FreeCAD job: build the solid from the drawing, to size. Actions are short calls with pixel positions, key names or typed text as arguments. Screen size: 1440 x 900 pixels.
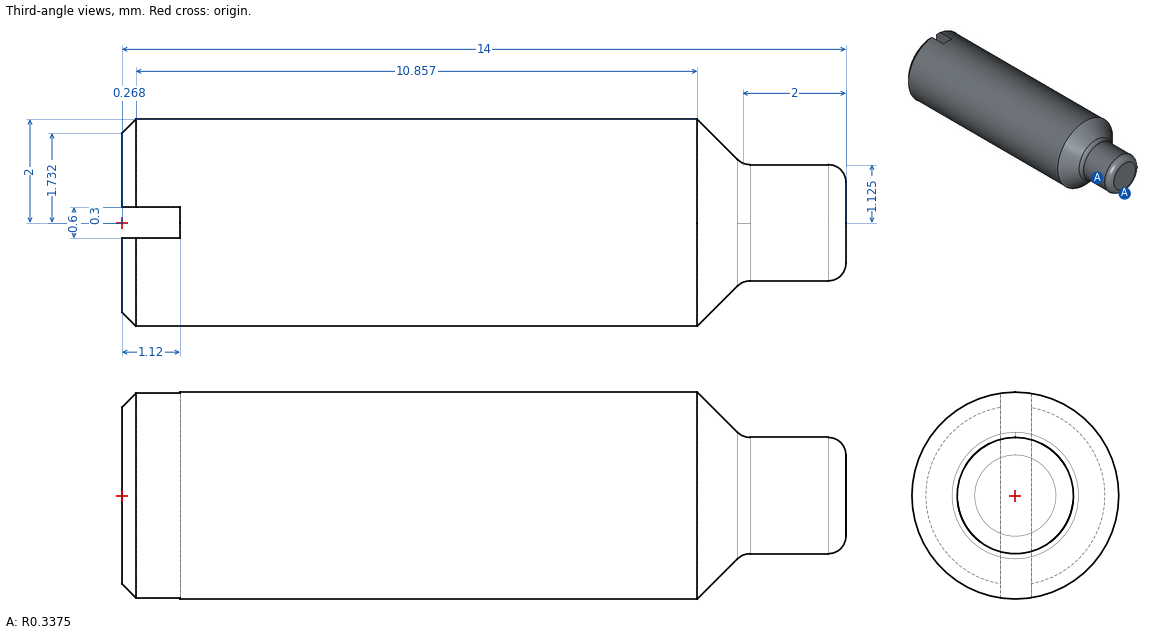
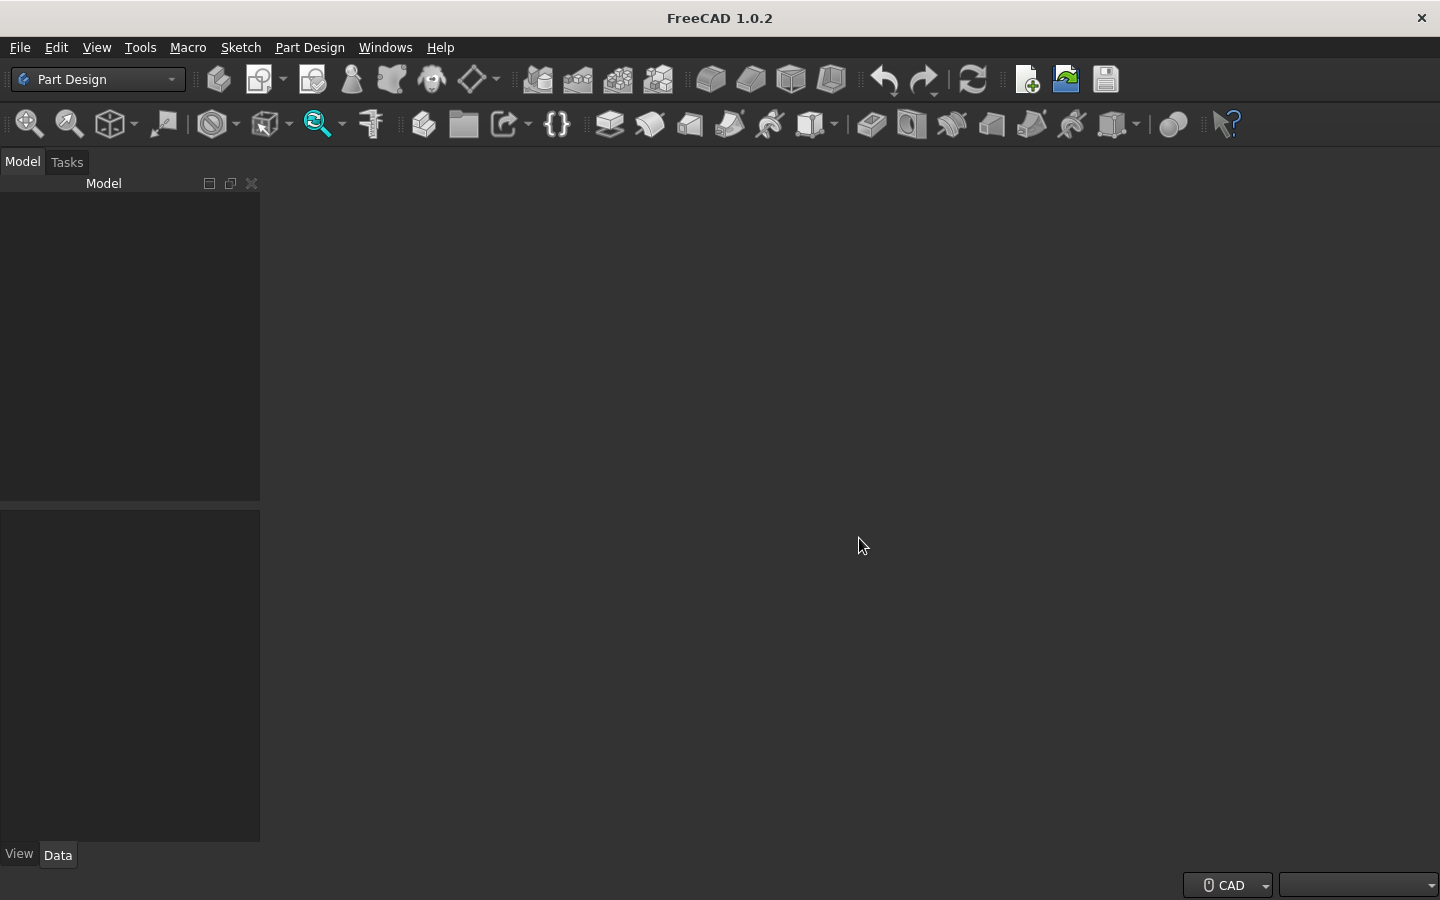
key(ctrl+n)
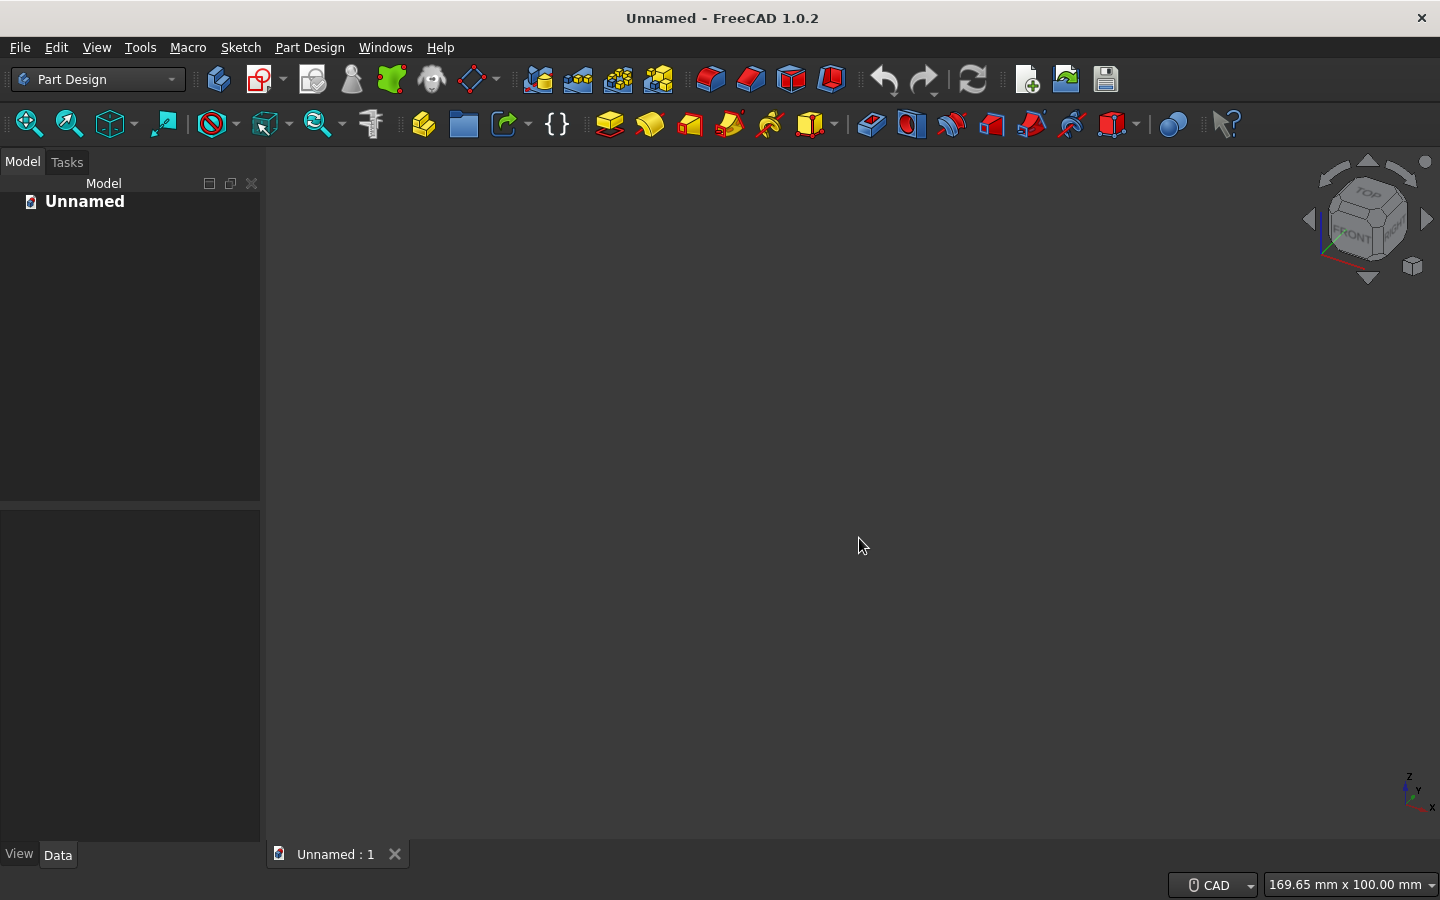
click(260, 80)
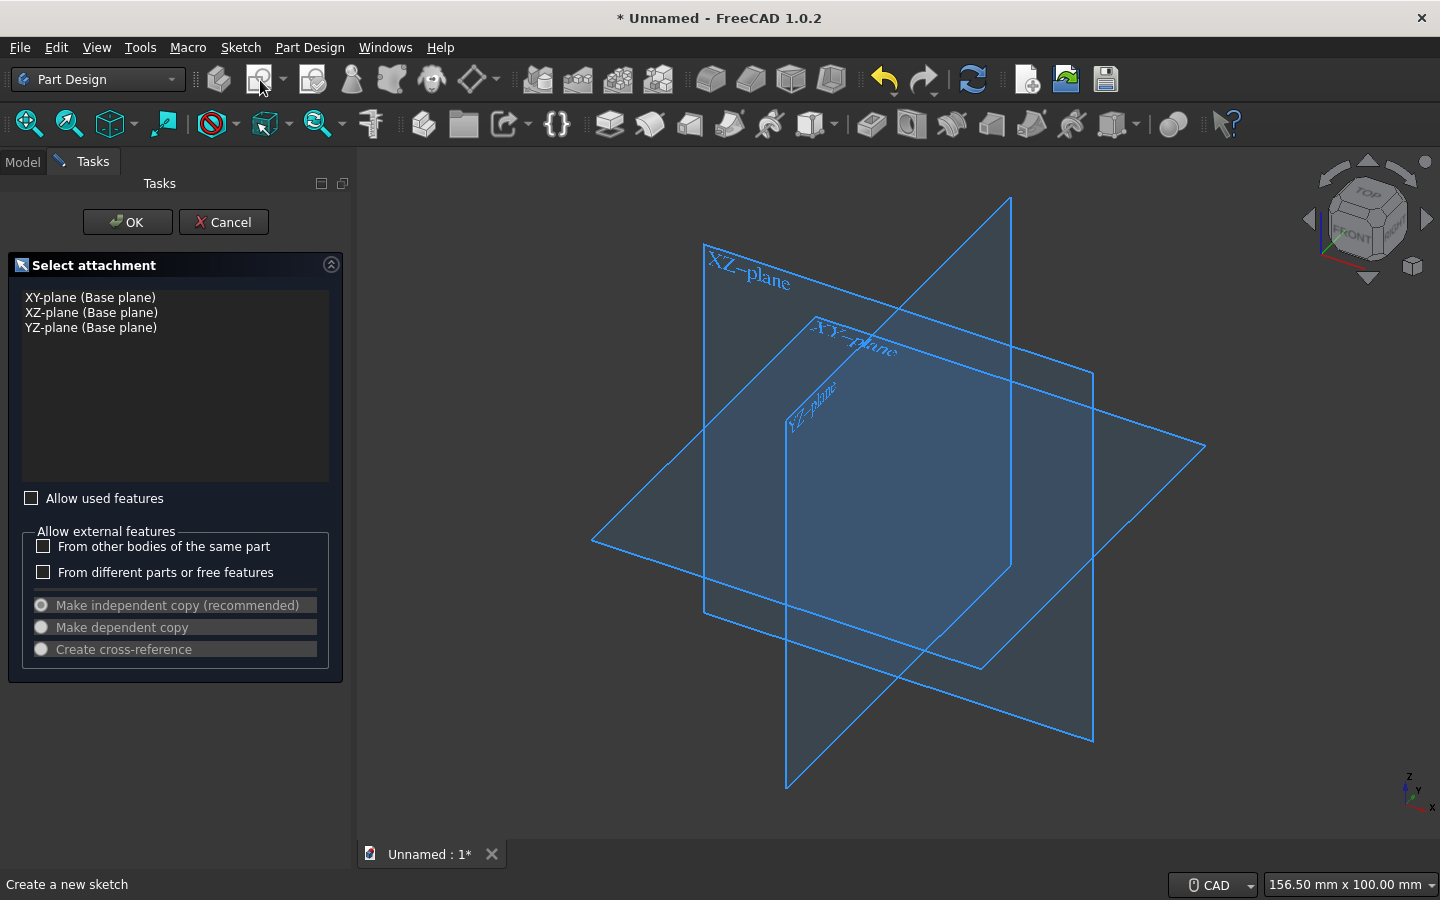
click(82, 298)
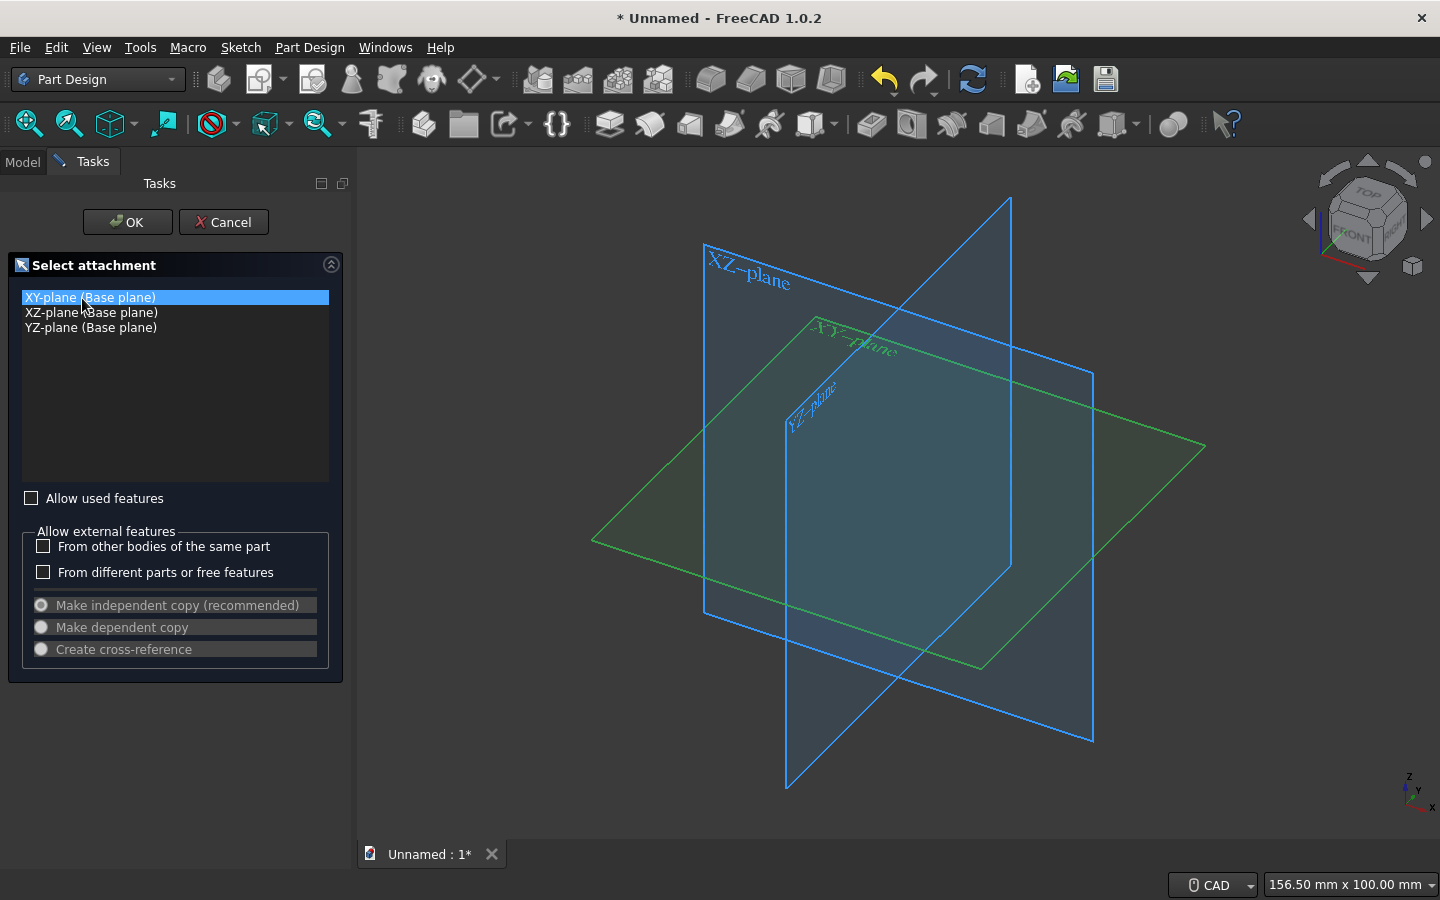
click(128, 222)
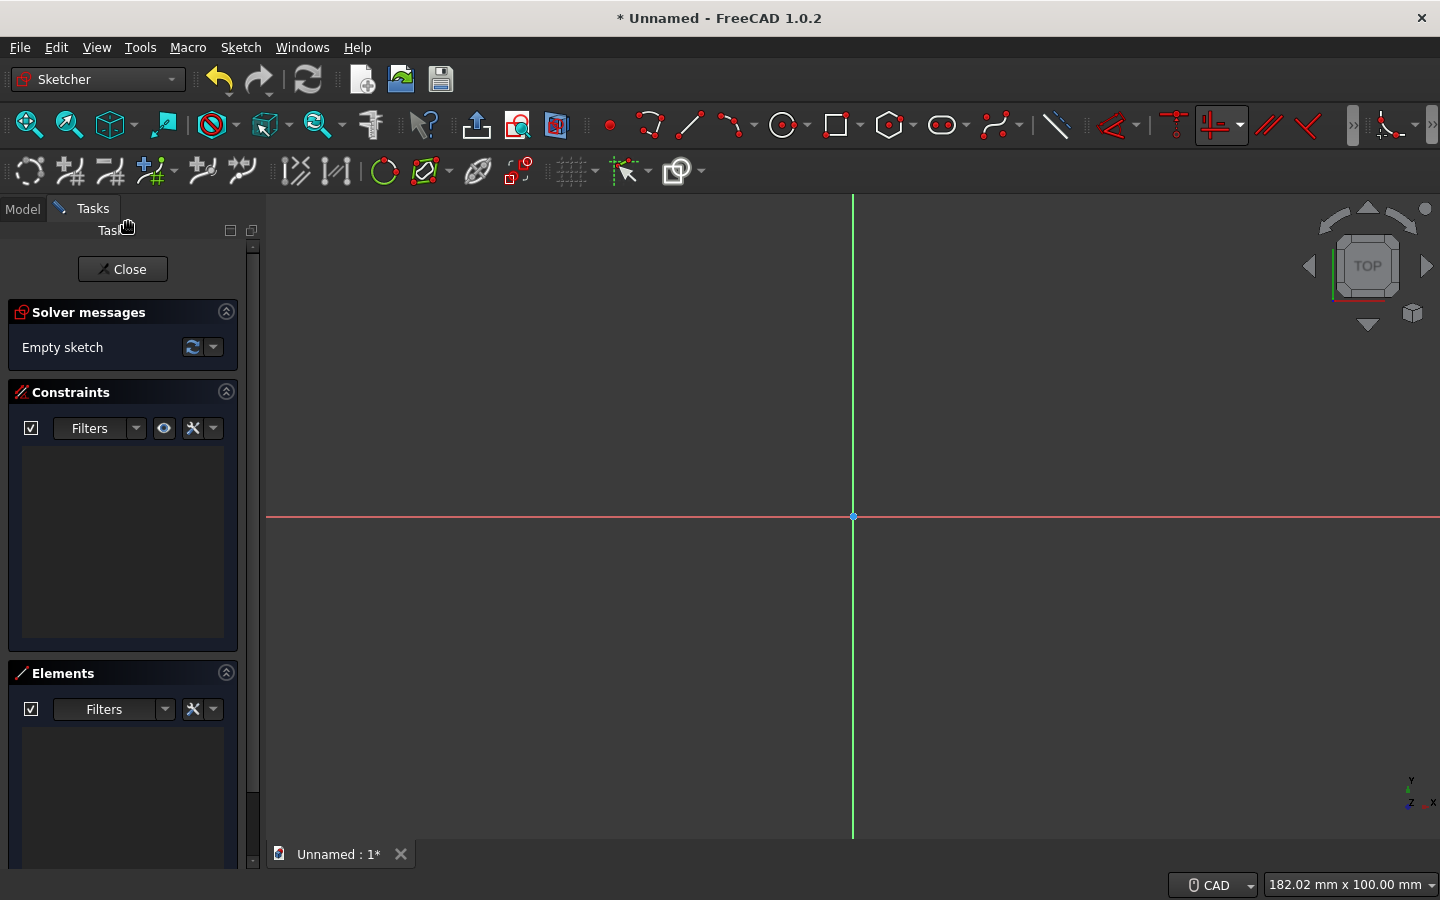
scroll(916, 509, up, 10)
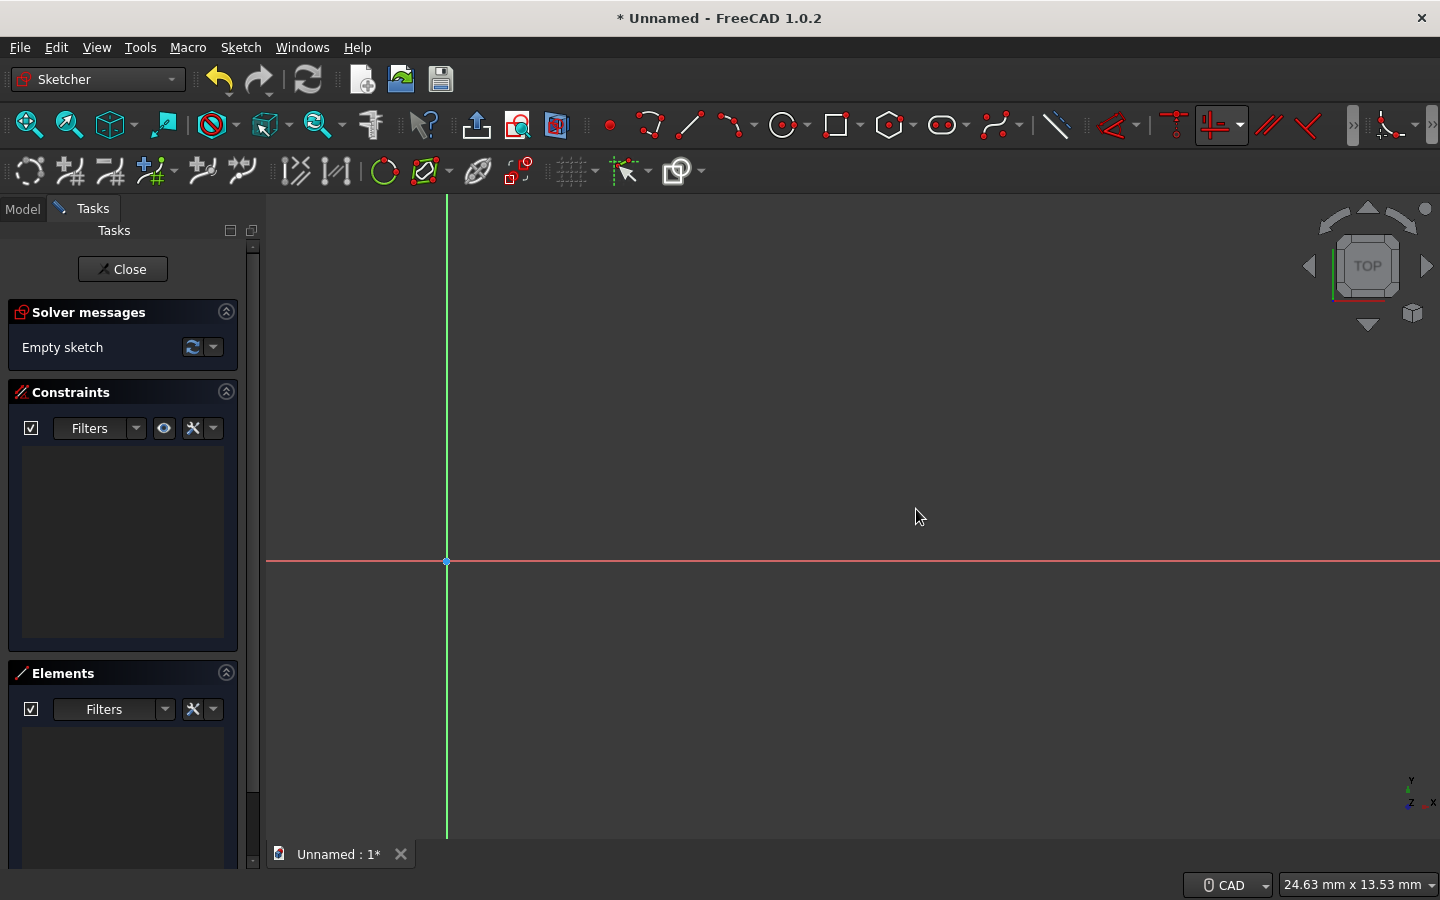
key(g)
key(m)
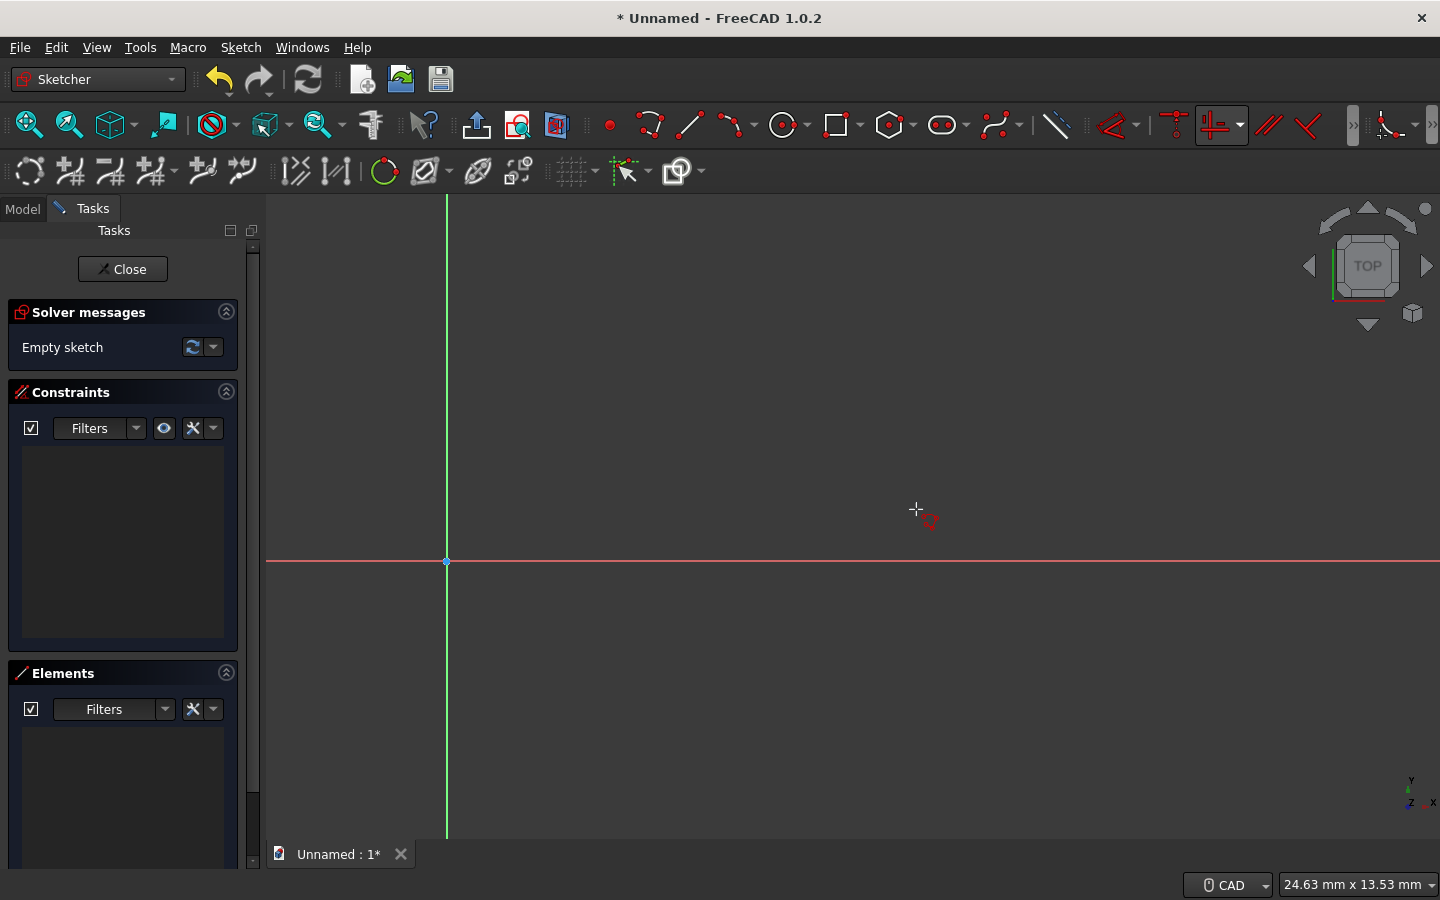
click(447, 561)
click(1114, 552)
click(1114, 508)
click(1019, 508)
click(977, 466)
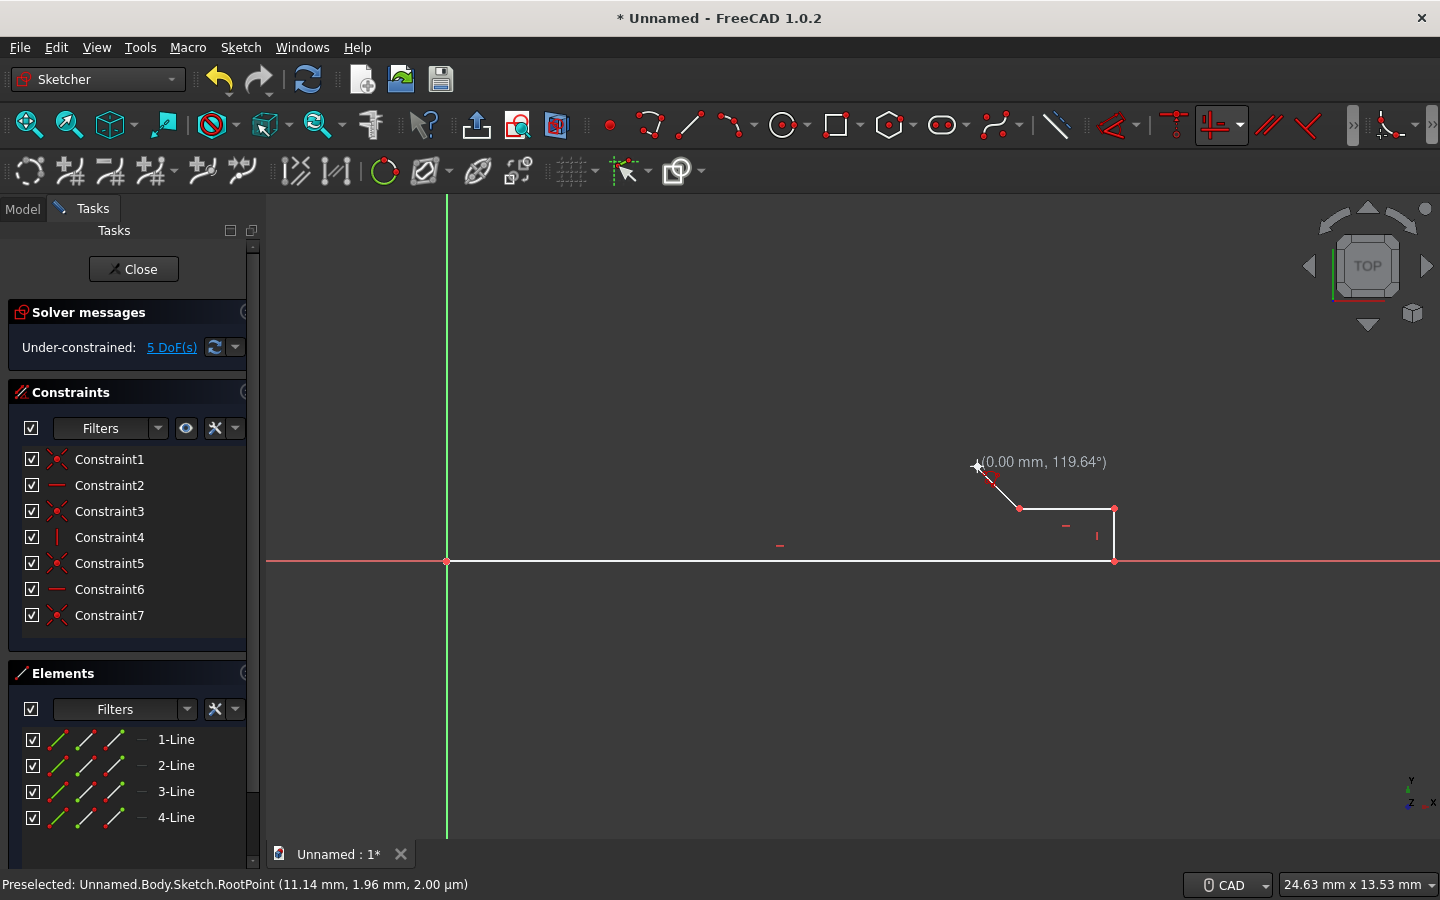
scroll(460, 466, up, 2)